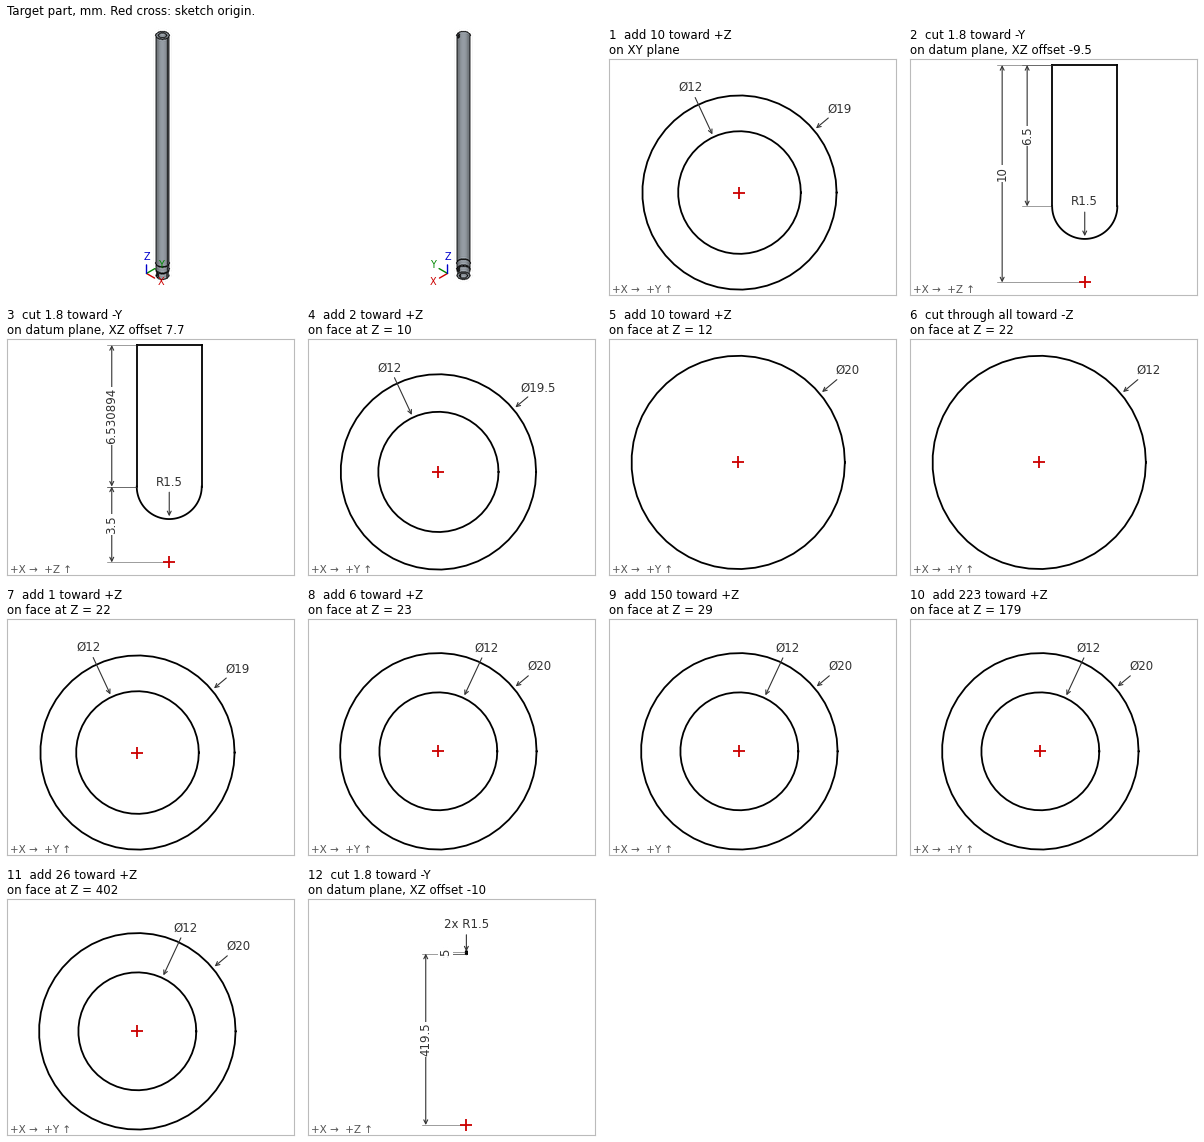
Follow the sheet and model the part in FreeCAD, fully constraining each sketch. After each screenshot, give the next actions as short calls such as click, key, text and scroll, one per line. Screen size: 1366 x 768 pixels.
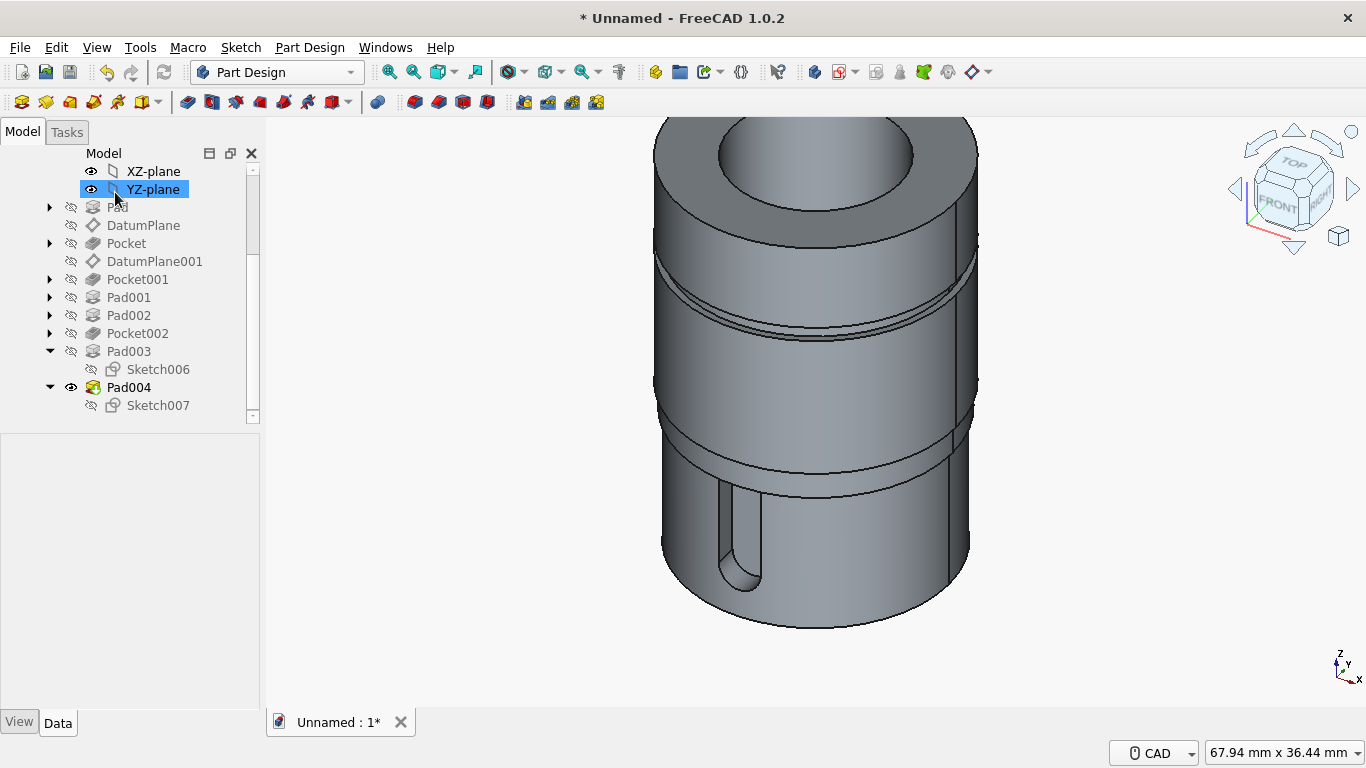
click(390, 72)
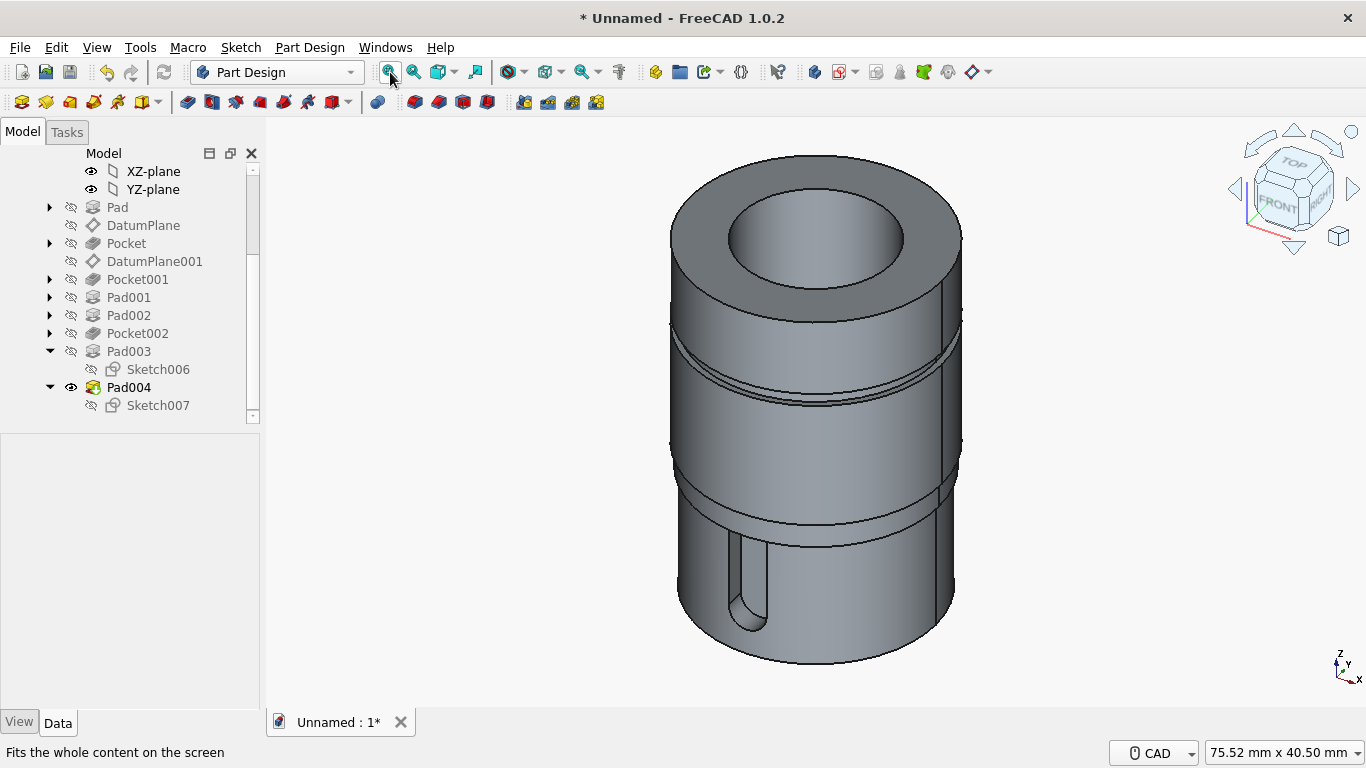
click(930, 221)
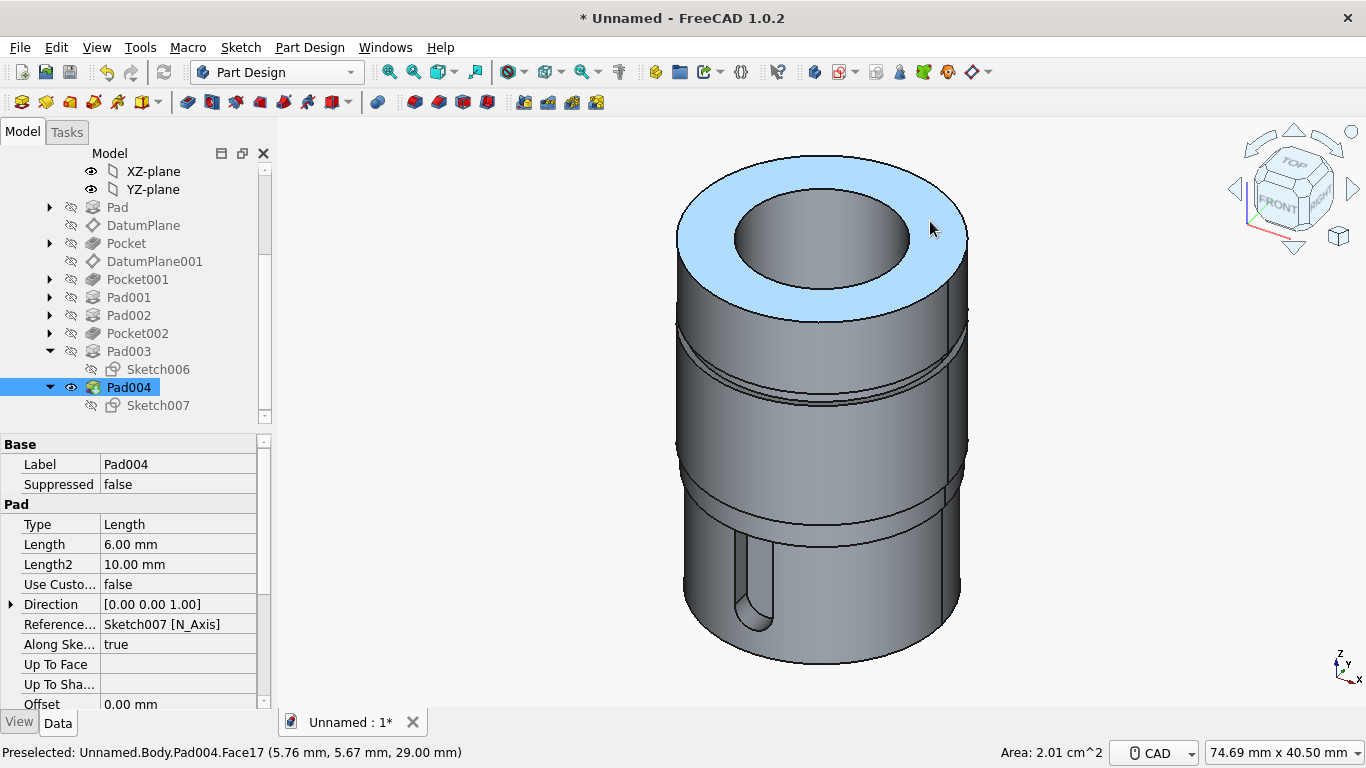
click(840, 72)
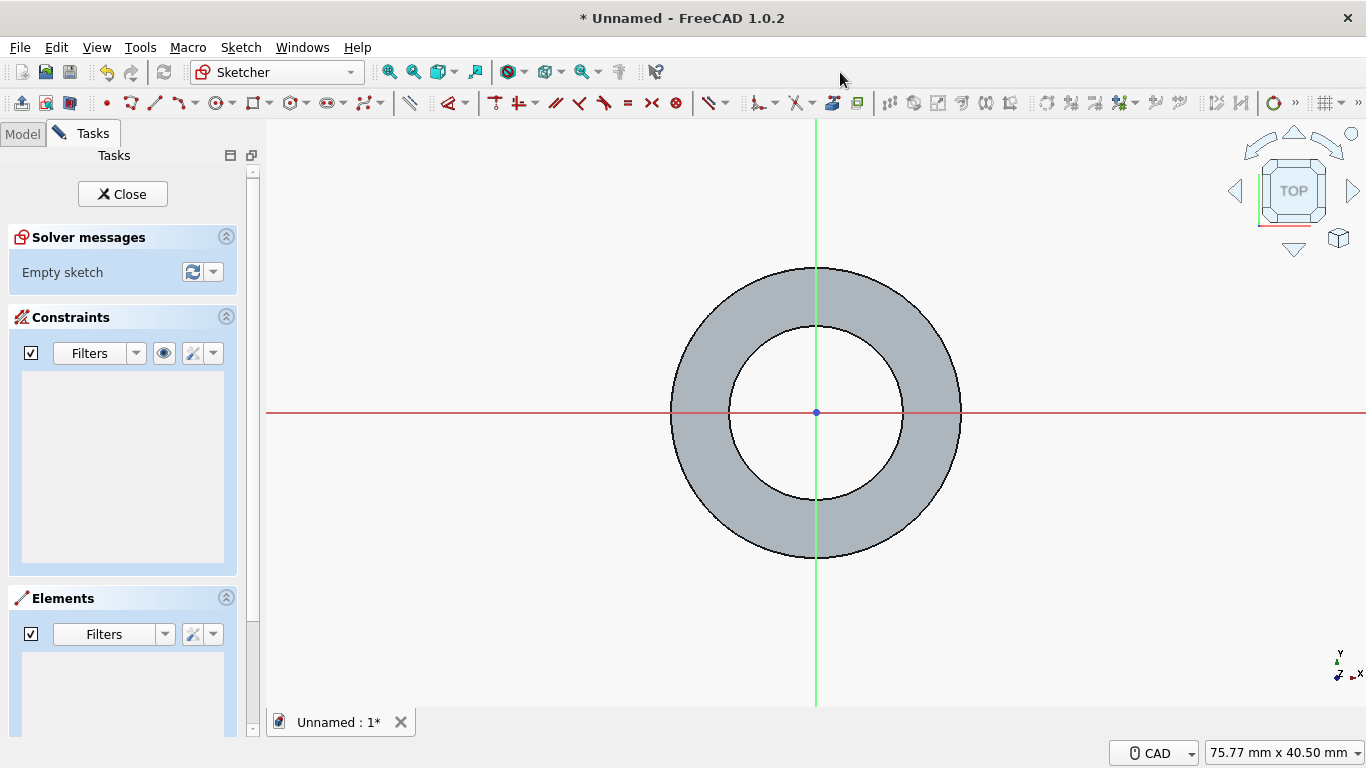
click(216, 104)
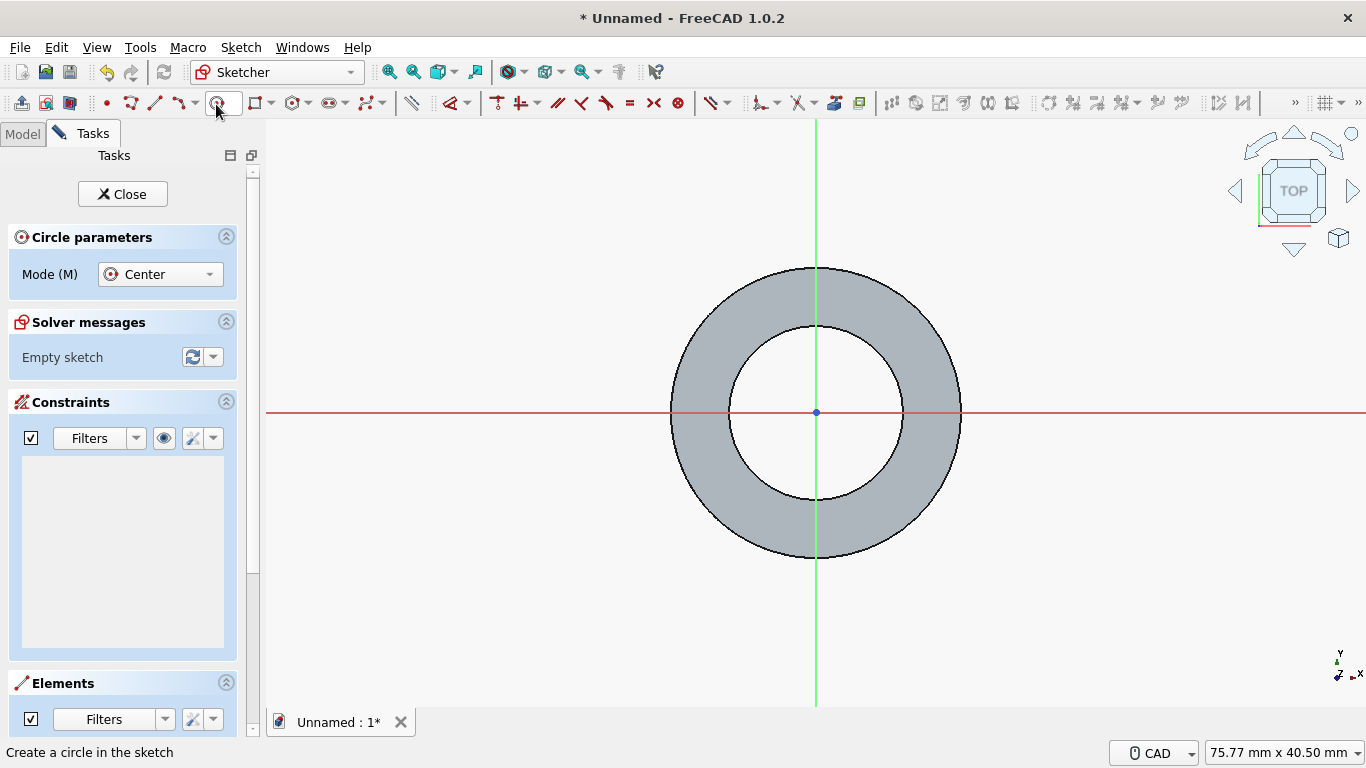
click(816, 413)
click(919, 310)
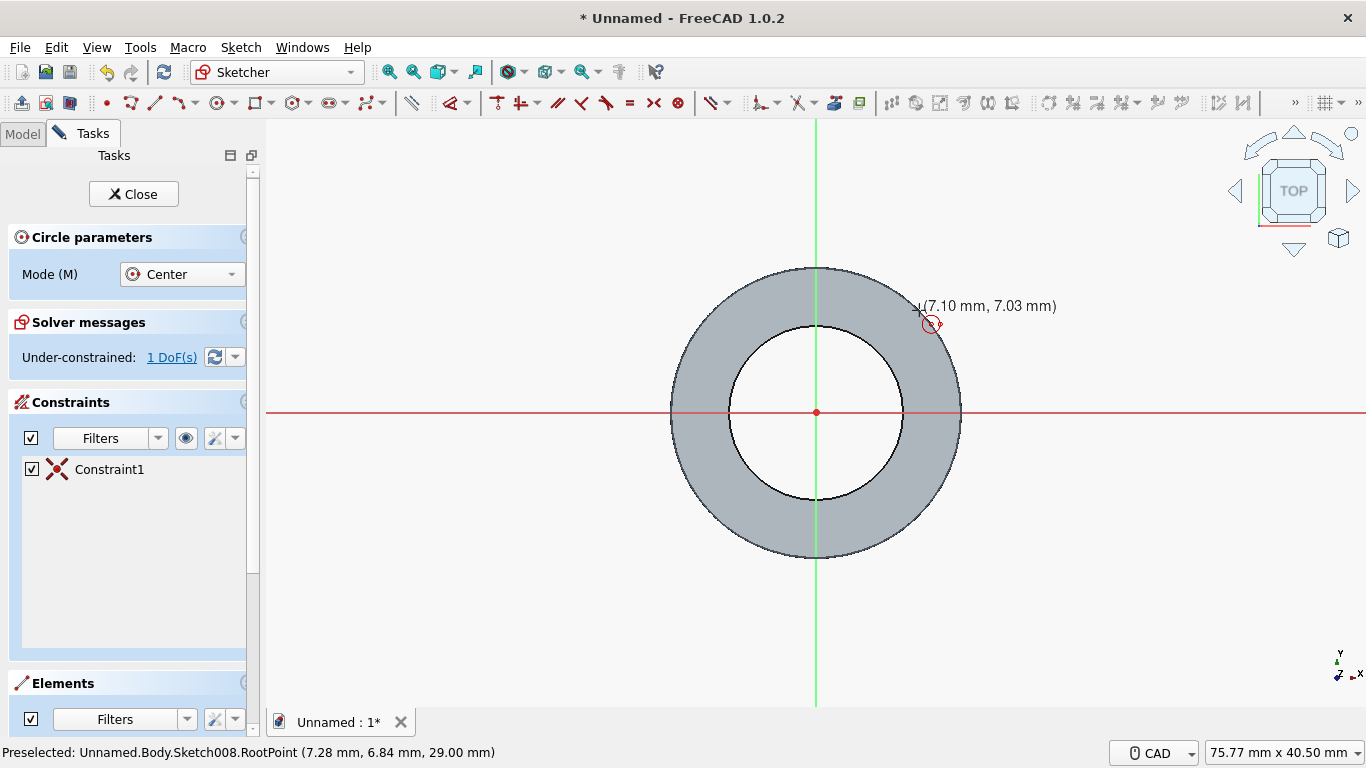
click(816, 413)
click(878, 351)
key(Escape)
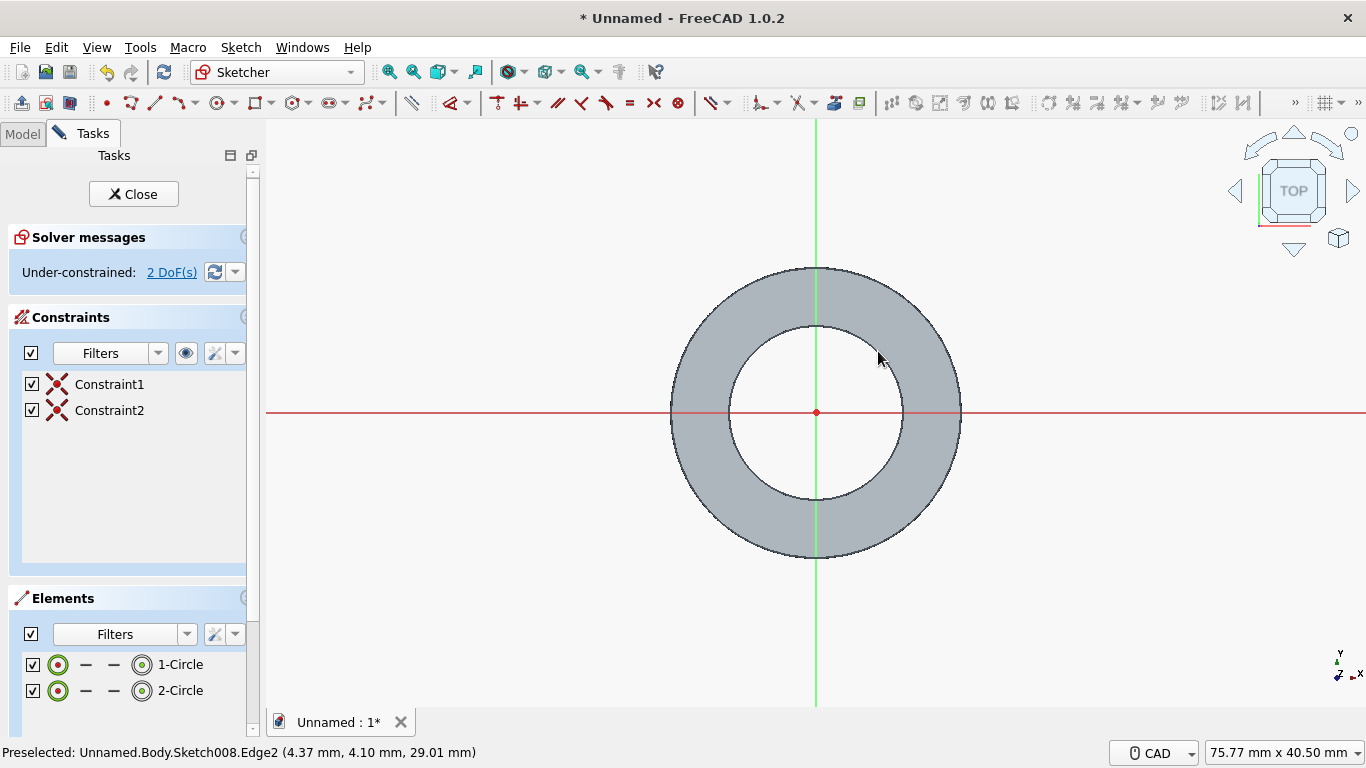
click(450, 104)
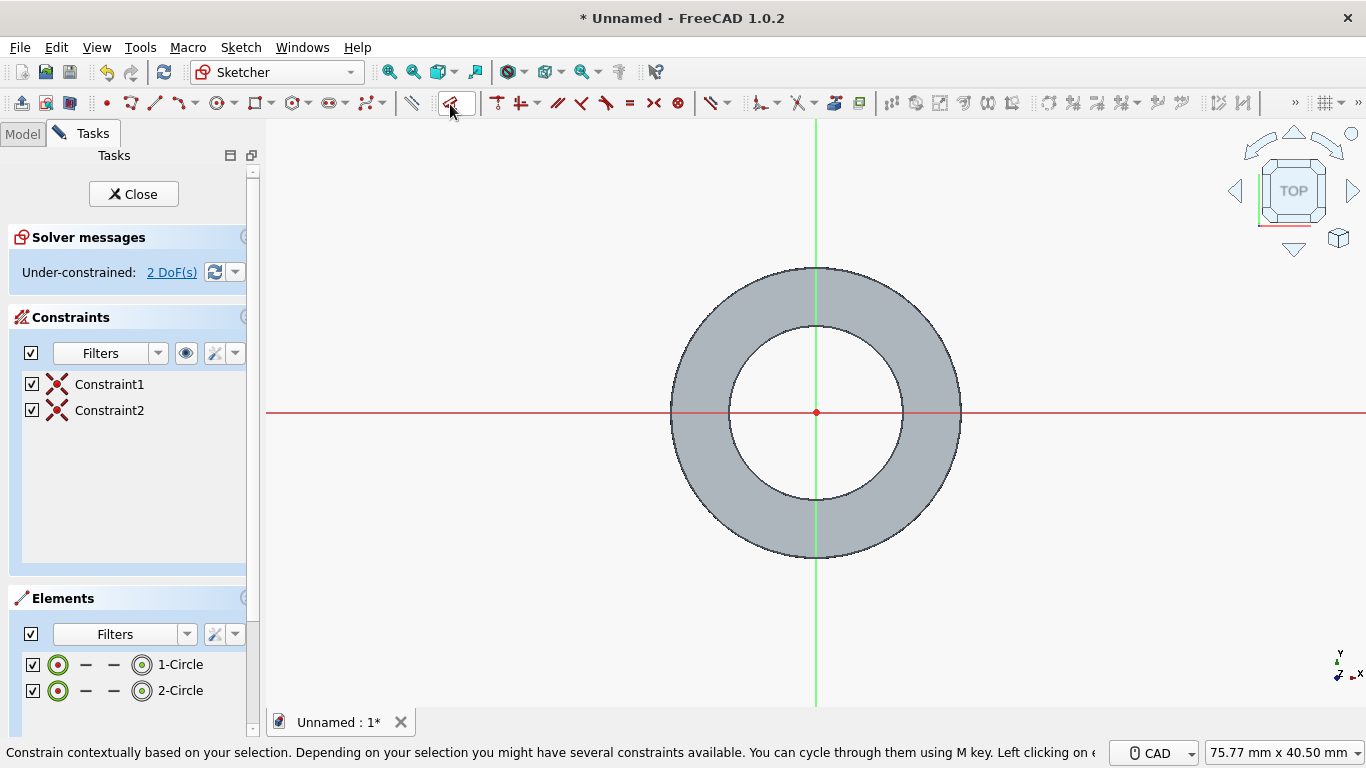
click(918, 310)
click(941, 287)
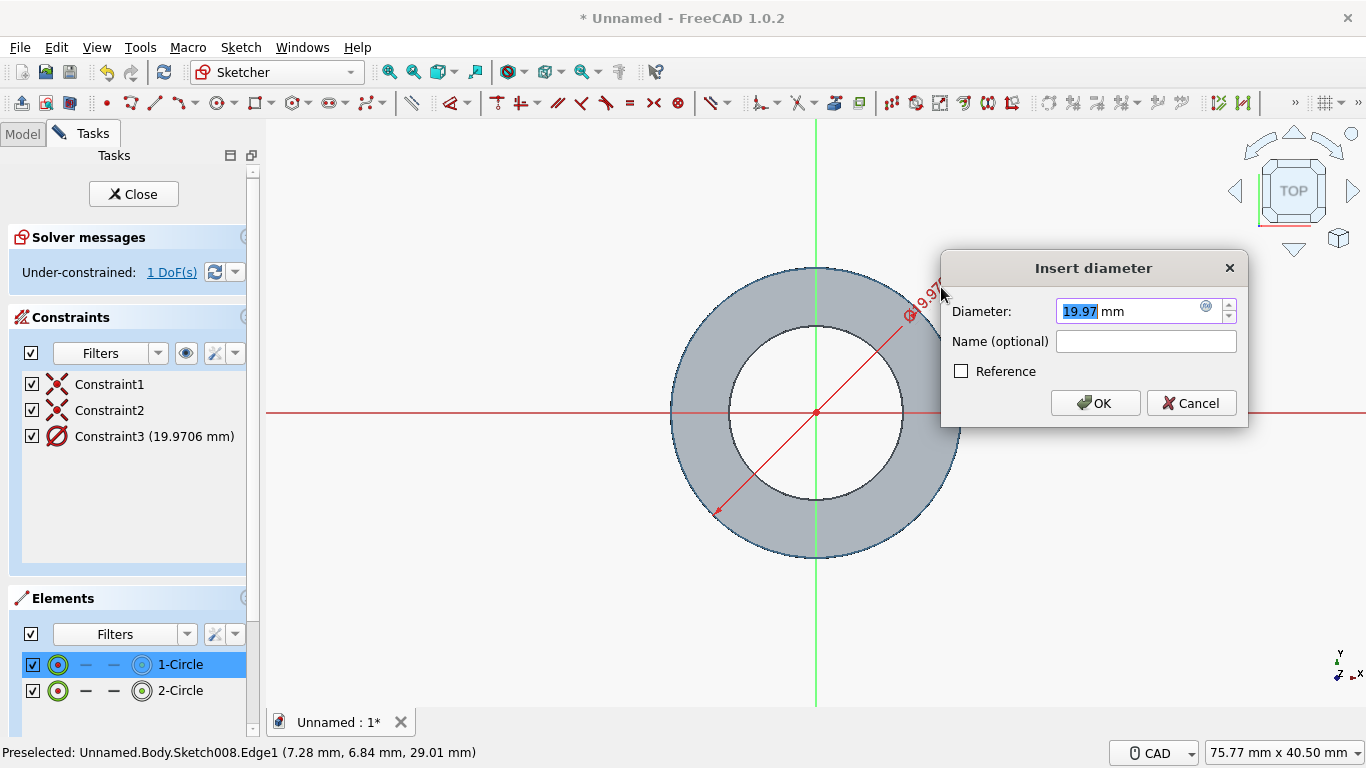
text(20)
key(Return)